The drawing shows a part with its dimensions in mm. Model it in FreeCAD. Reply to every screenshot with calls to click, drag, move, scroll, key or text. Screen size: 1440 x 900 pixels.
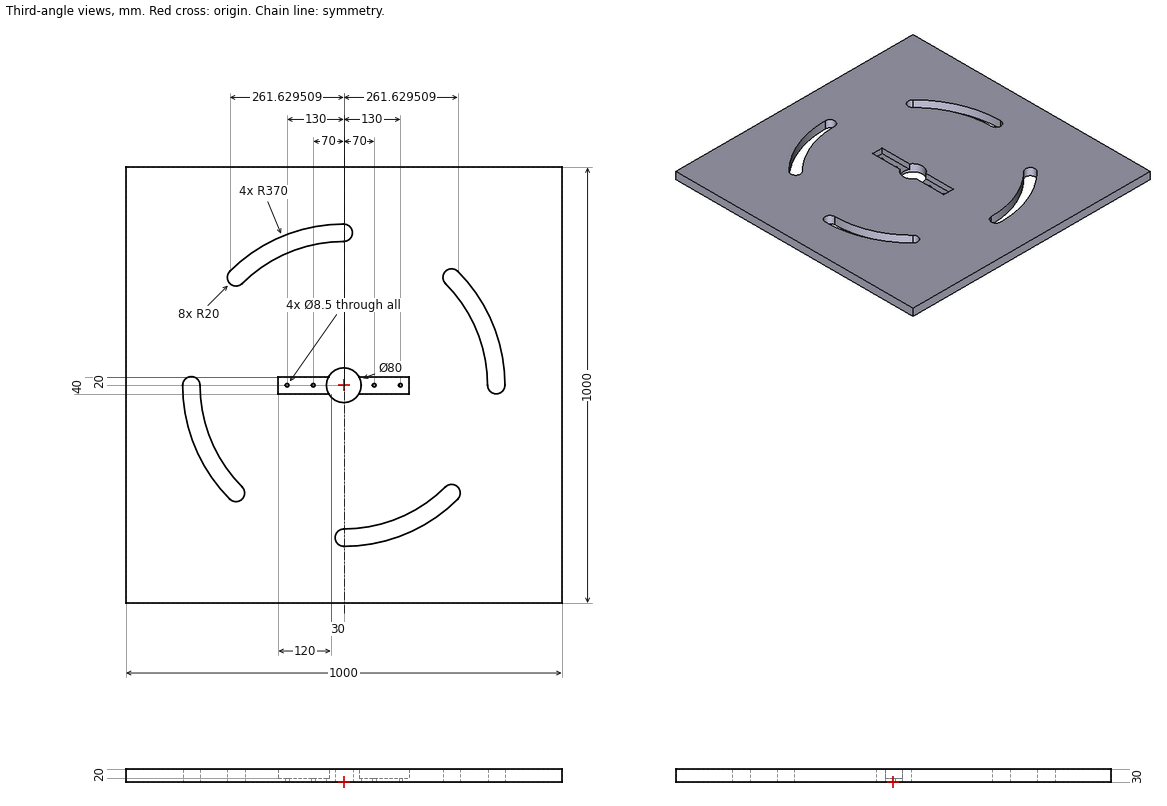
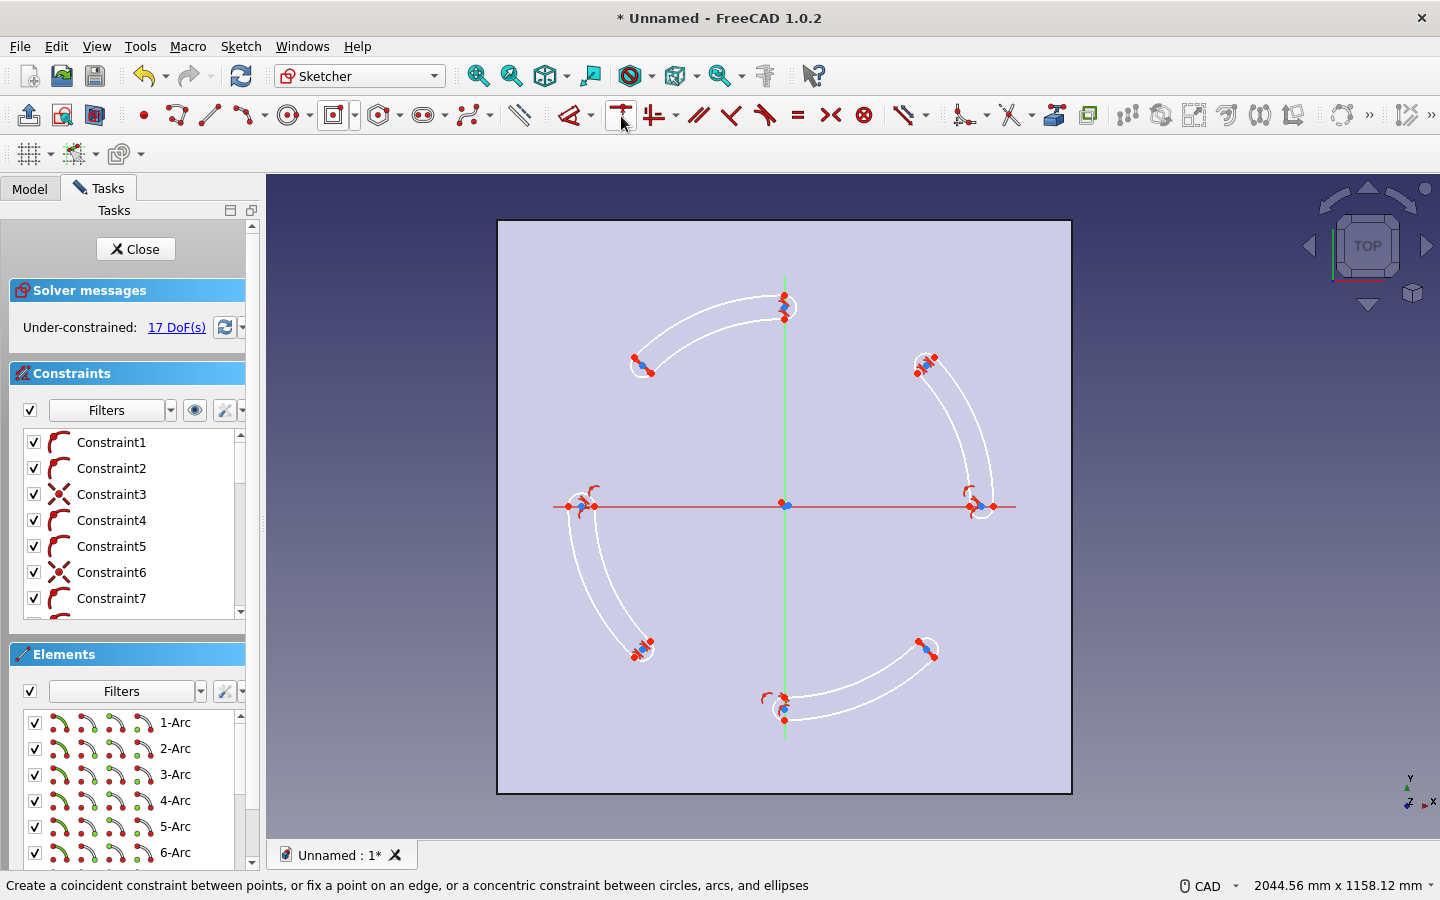
click(735, 301)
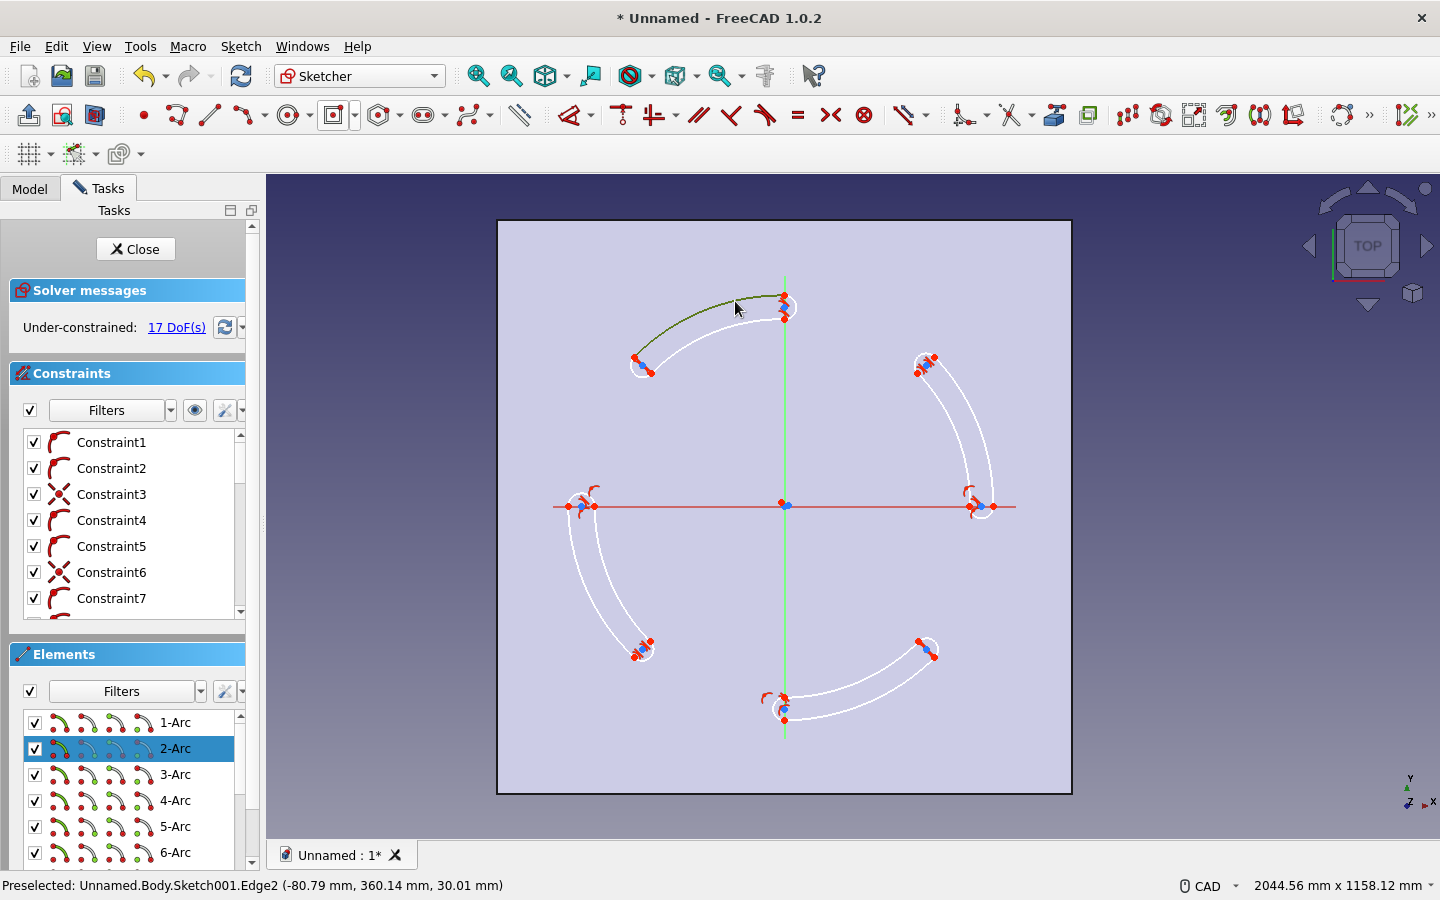
click(600, 551)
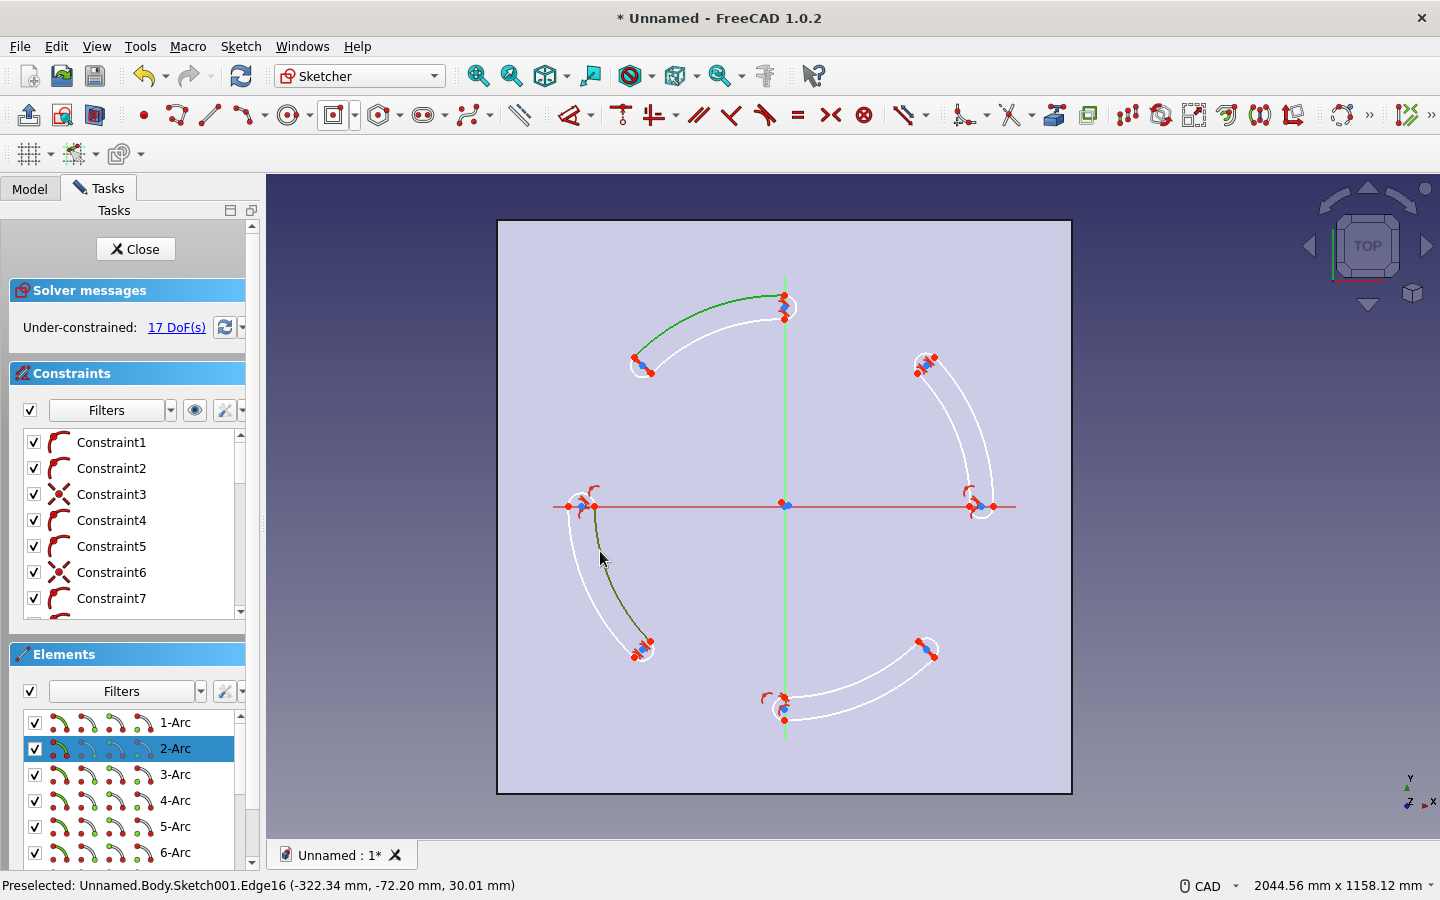
key(c)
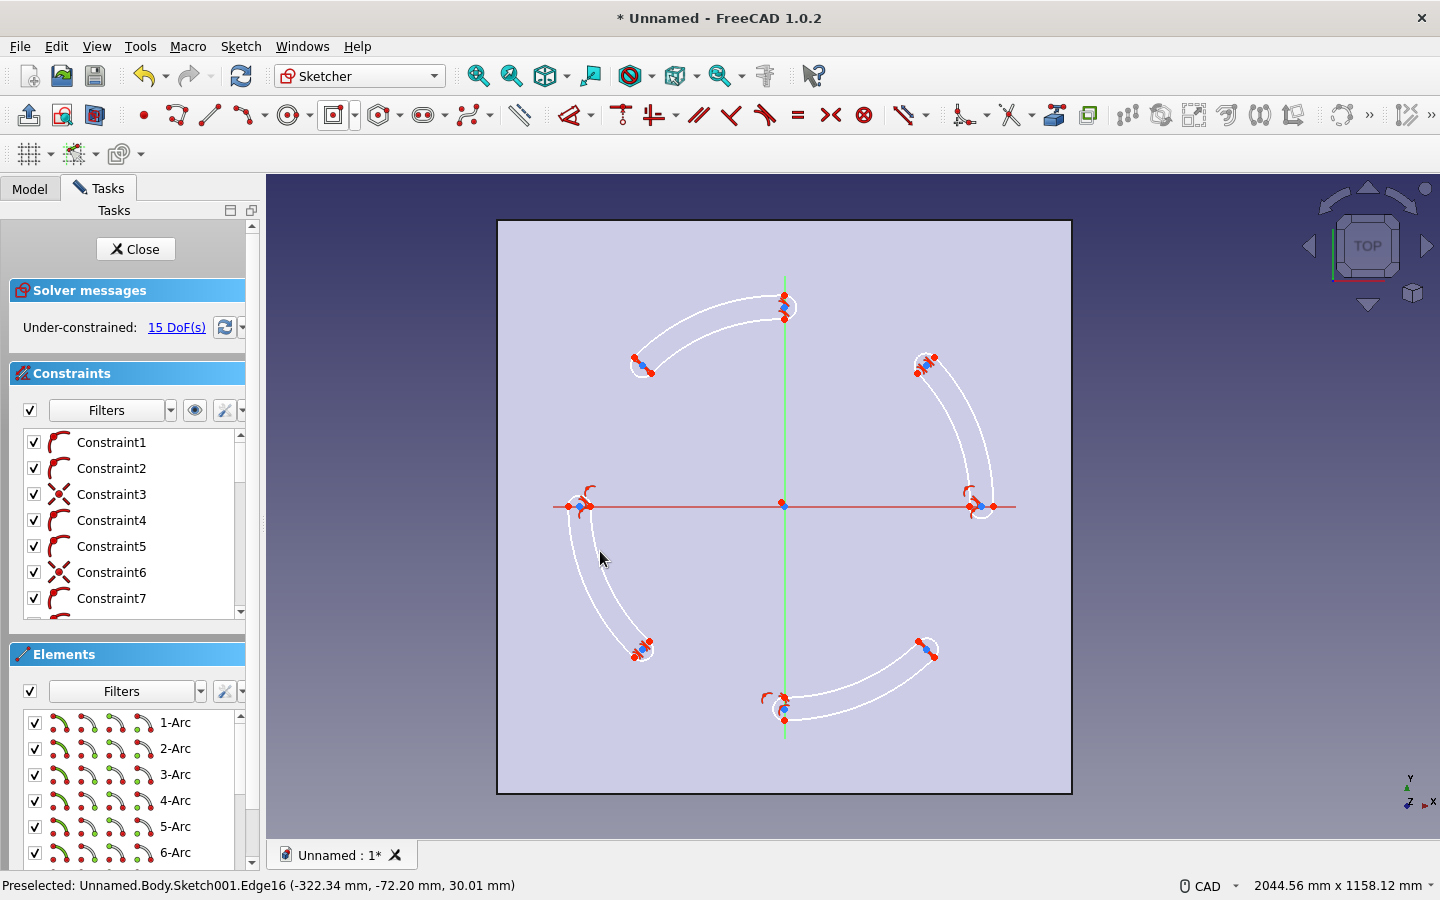
scroll(783, 505, up, 7)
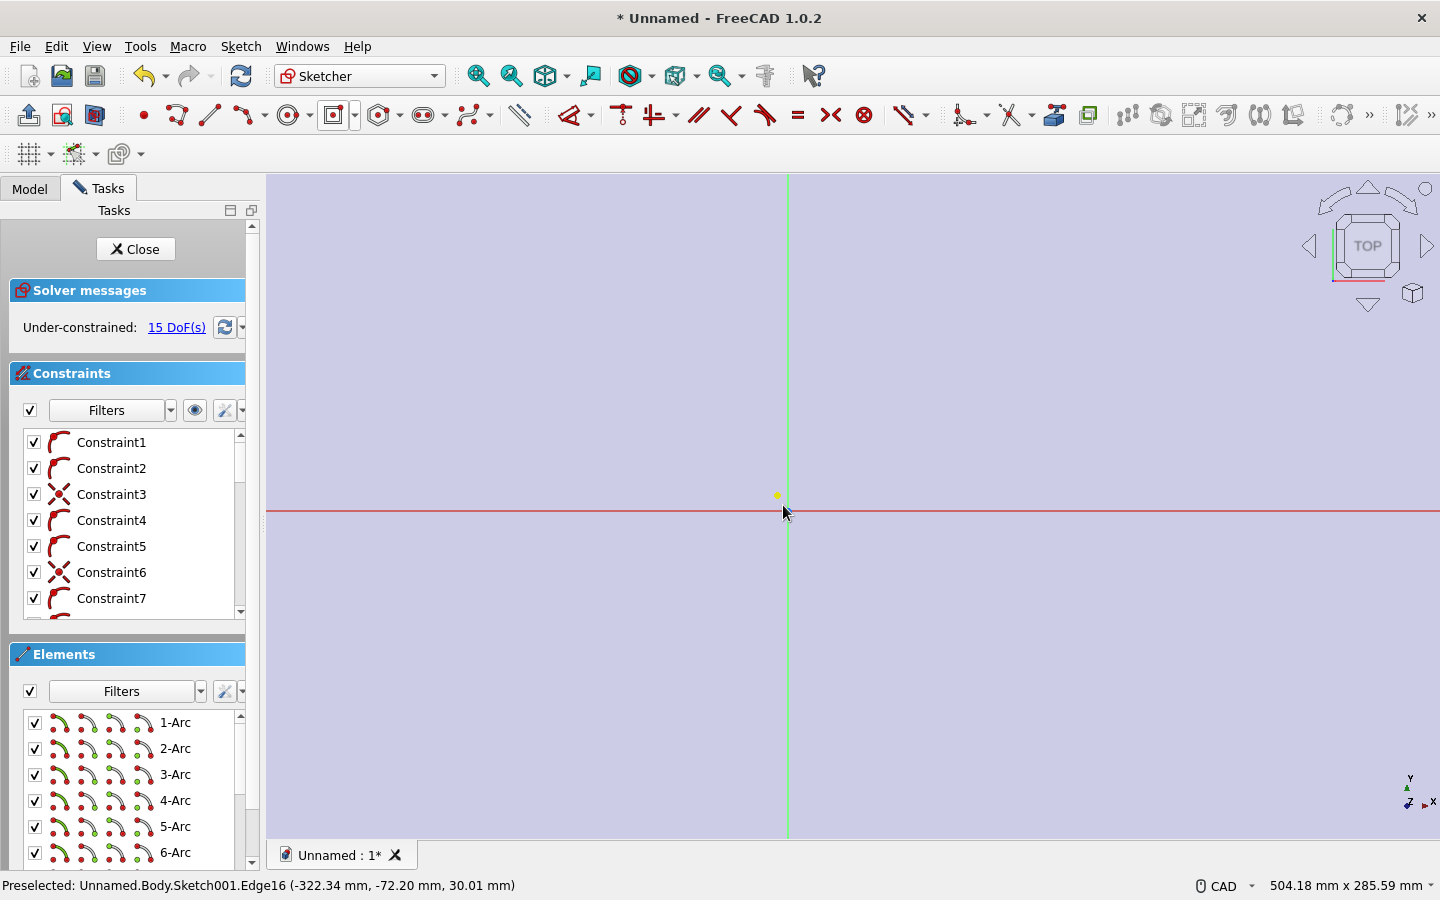
drag(767, 485, 798, 521)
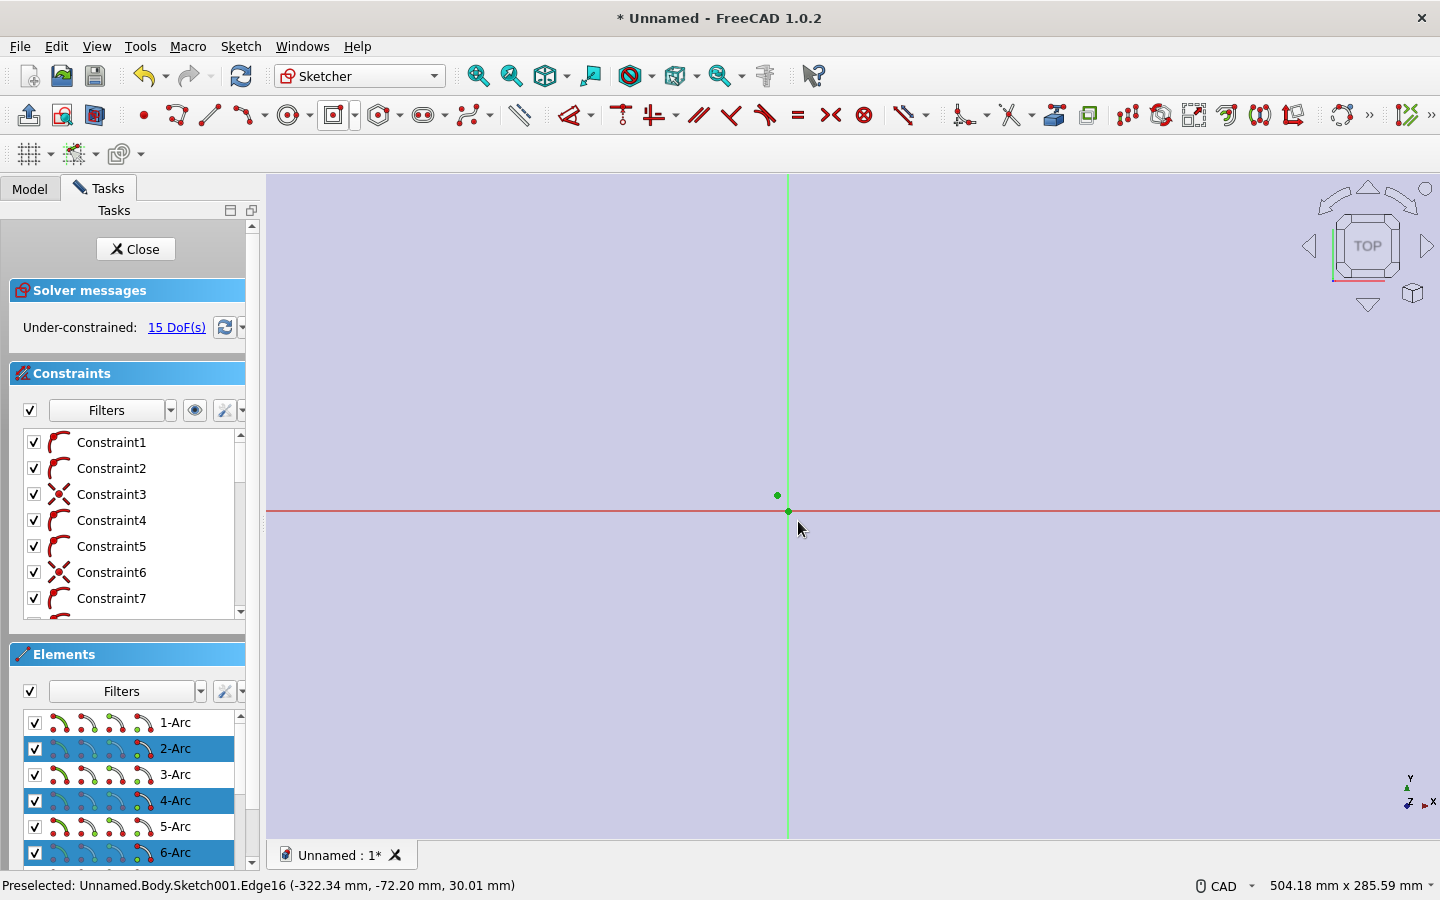
click(621, 116)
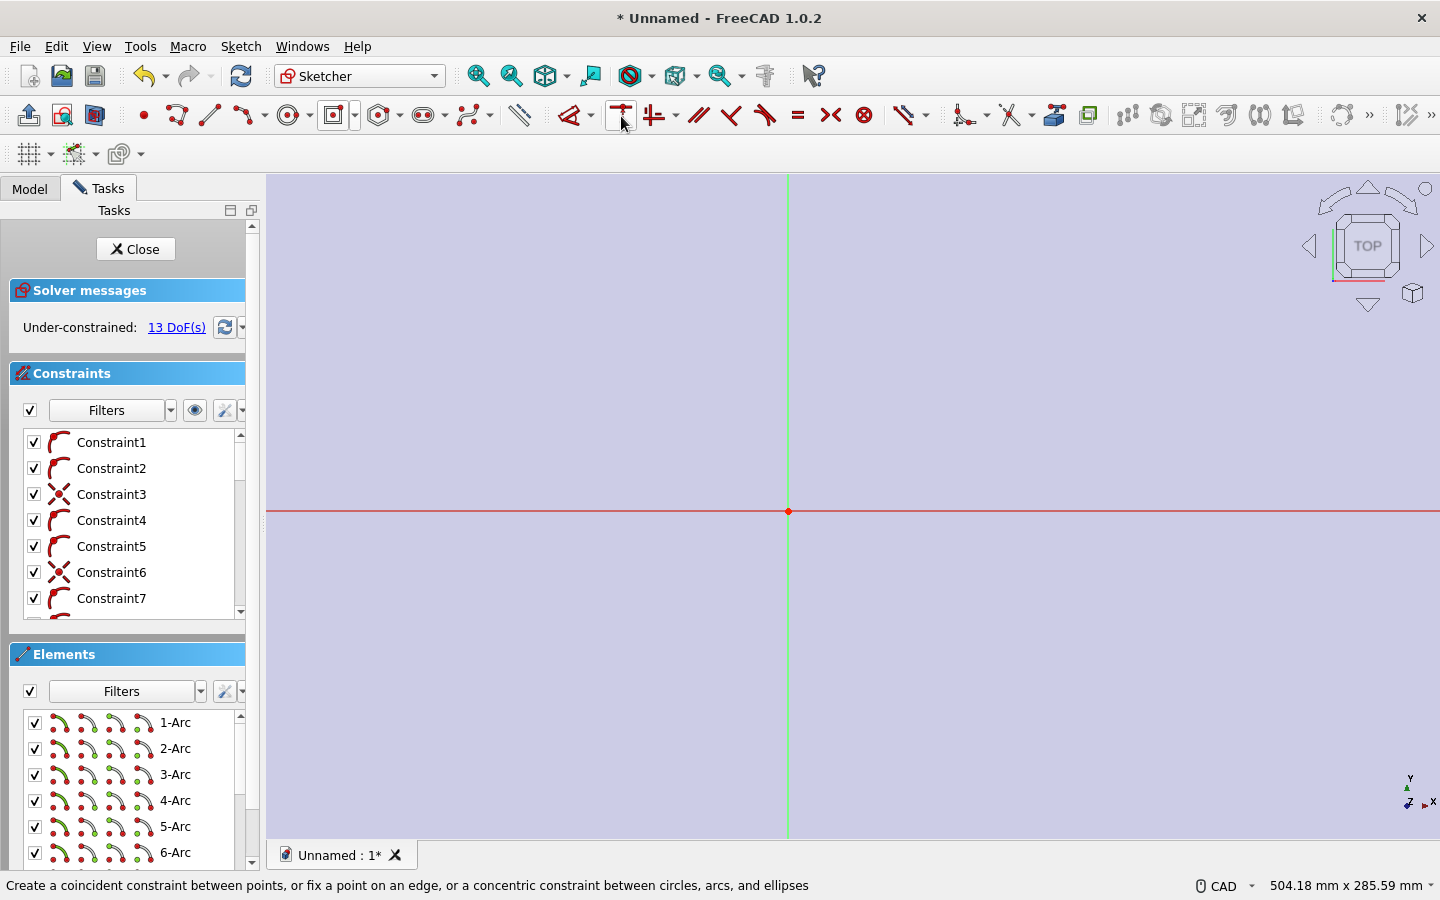
scroll(783, 505, down, 7)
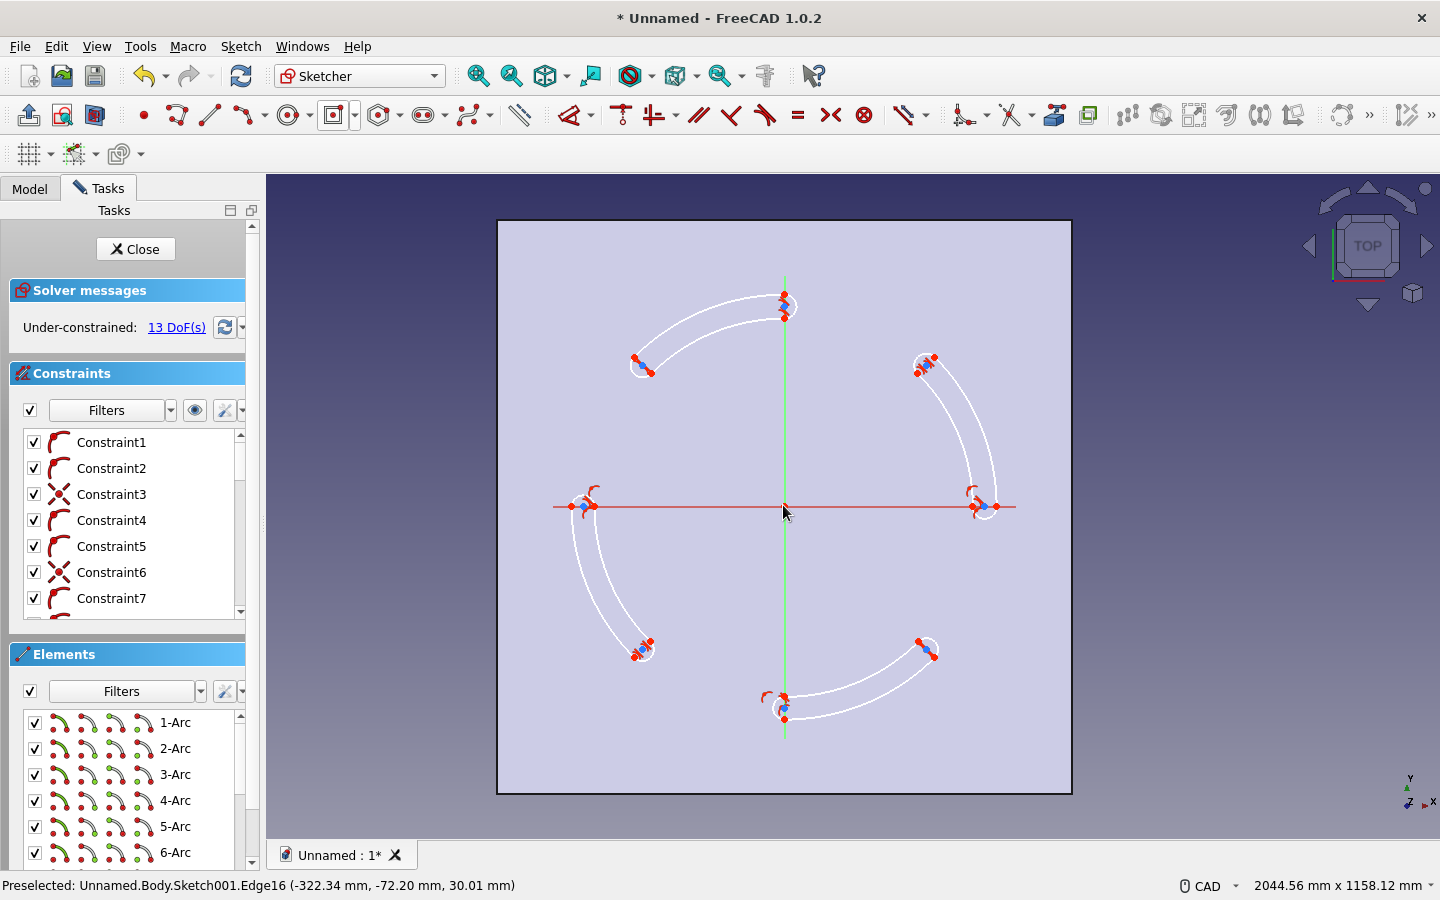
scroll(794, 314, up, 2)